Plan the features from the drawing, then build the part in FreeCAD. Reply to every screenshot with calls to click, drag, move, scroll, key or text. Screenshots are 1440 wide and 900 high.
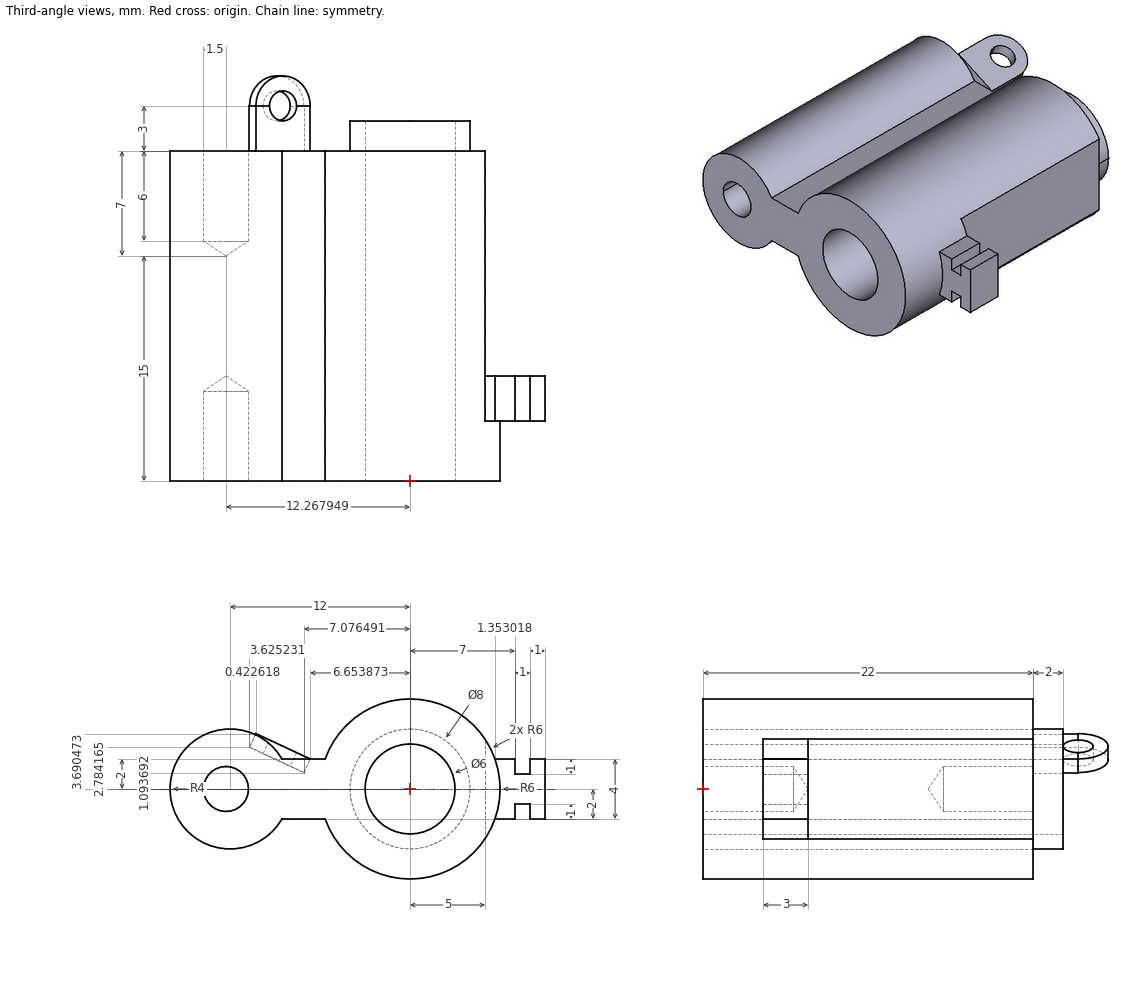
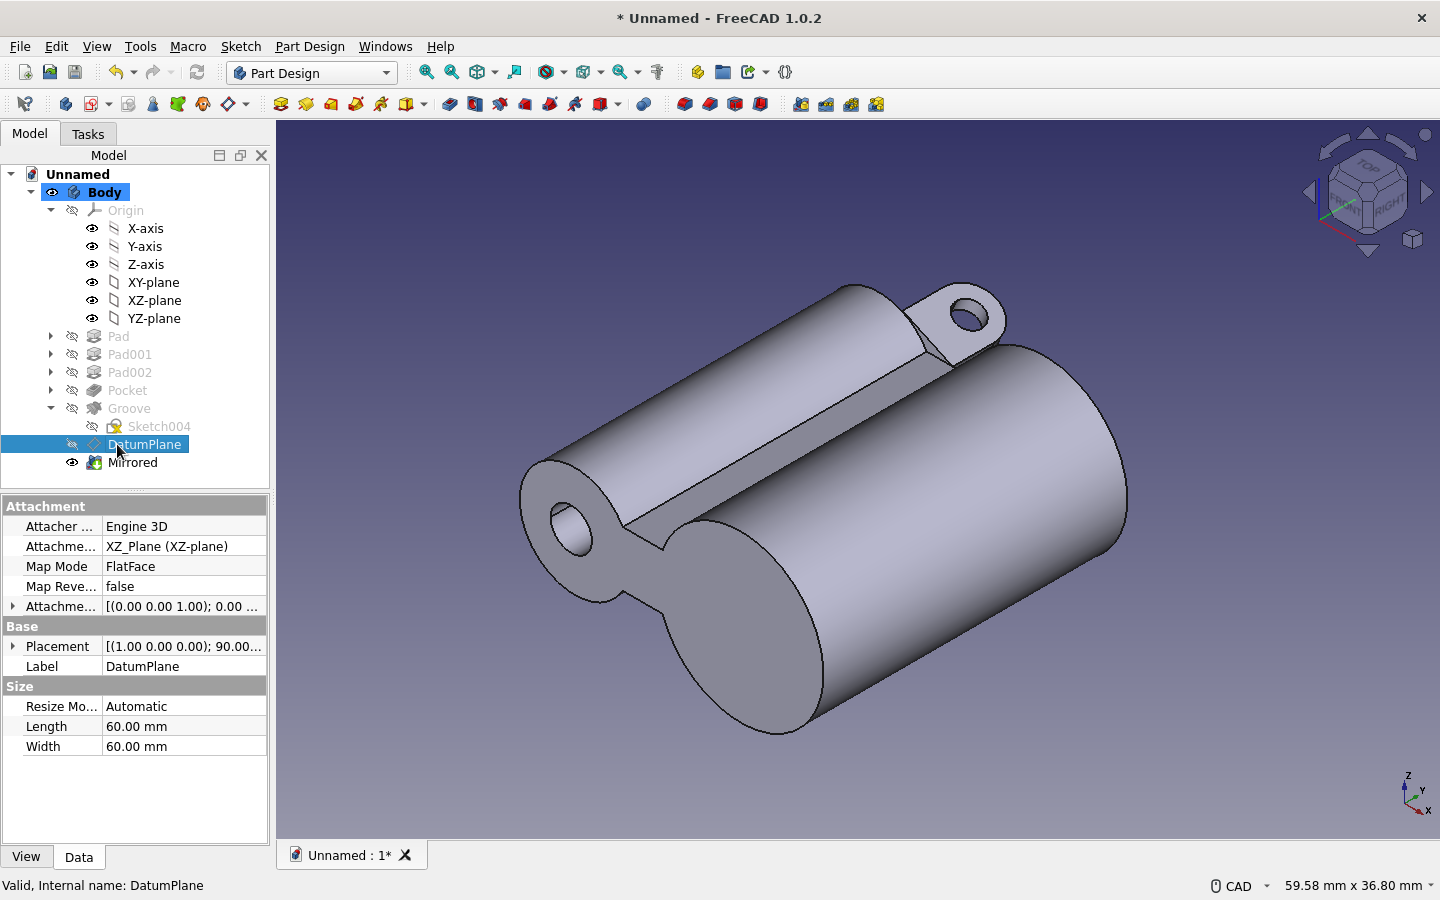
key(4)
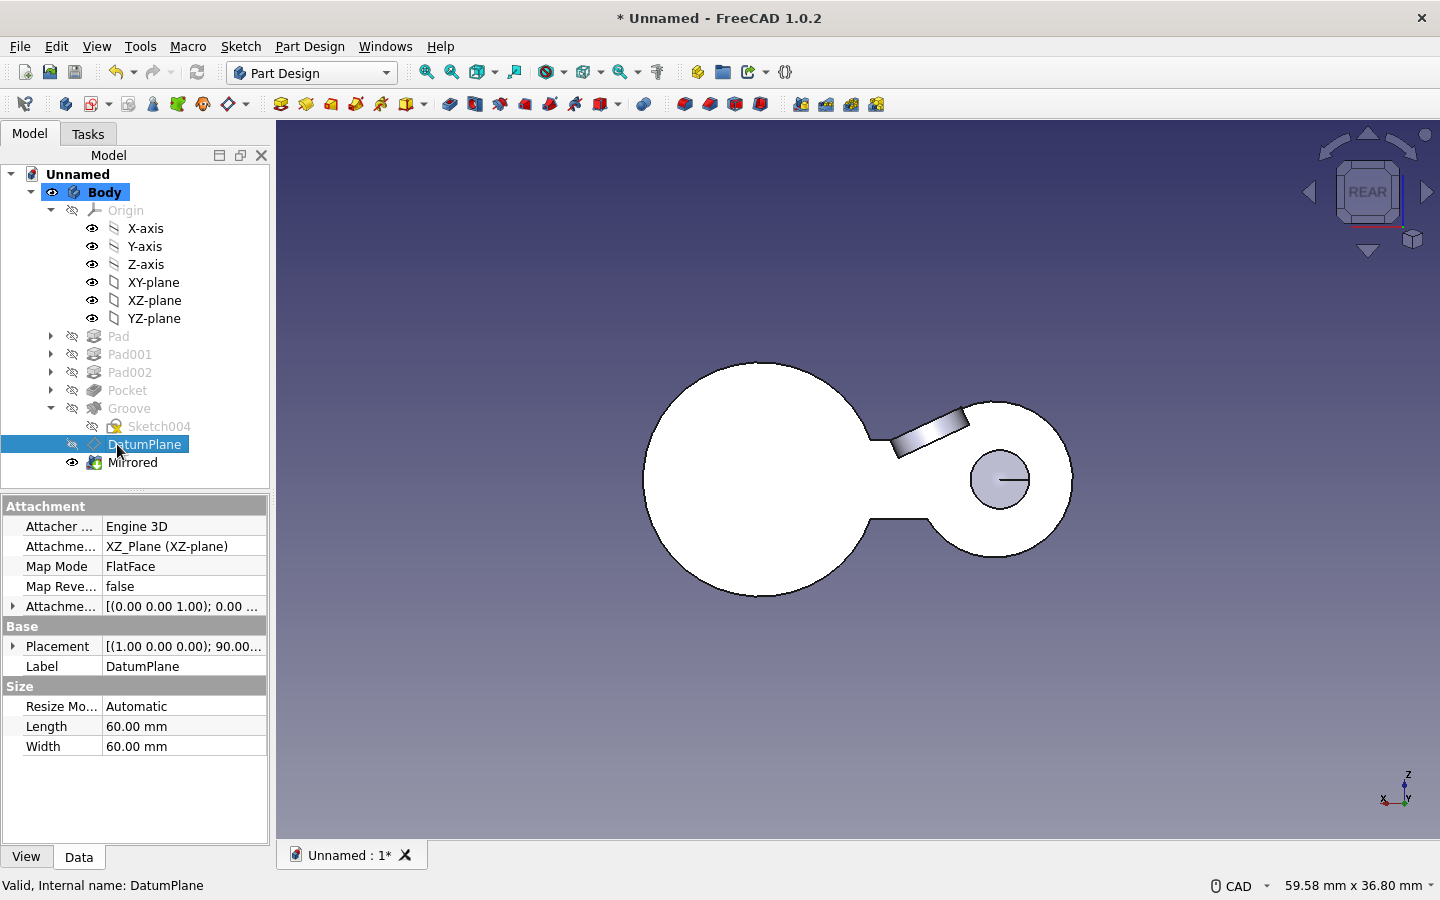
click(427, 72)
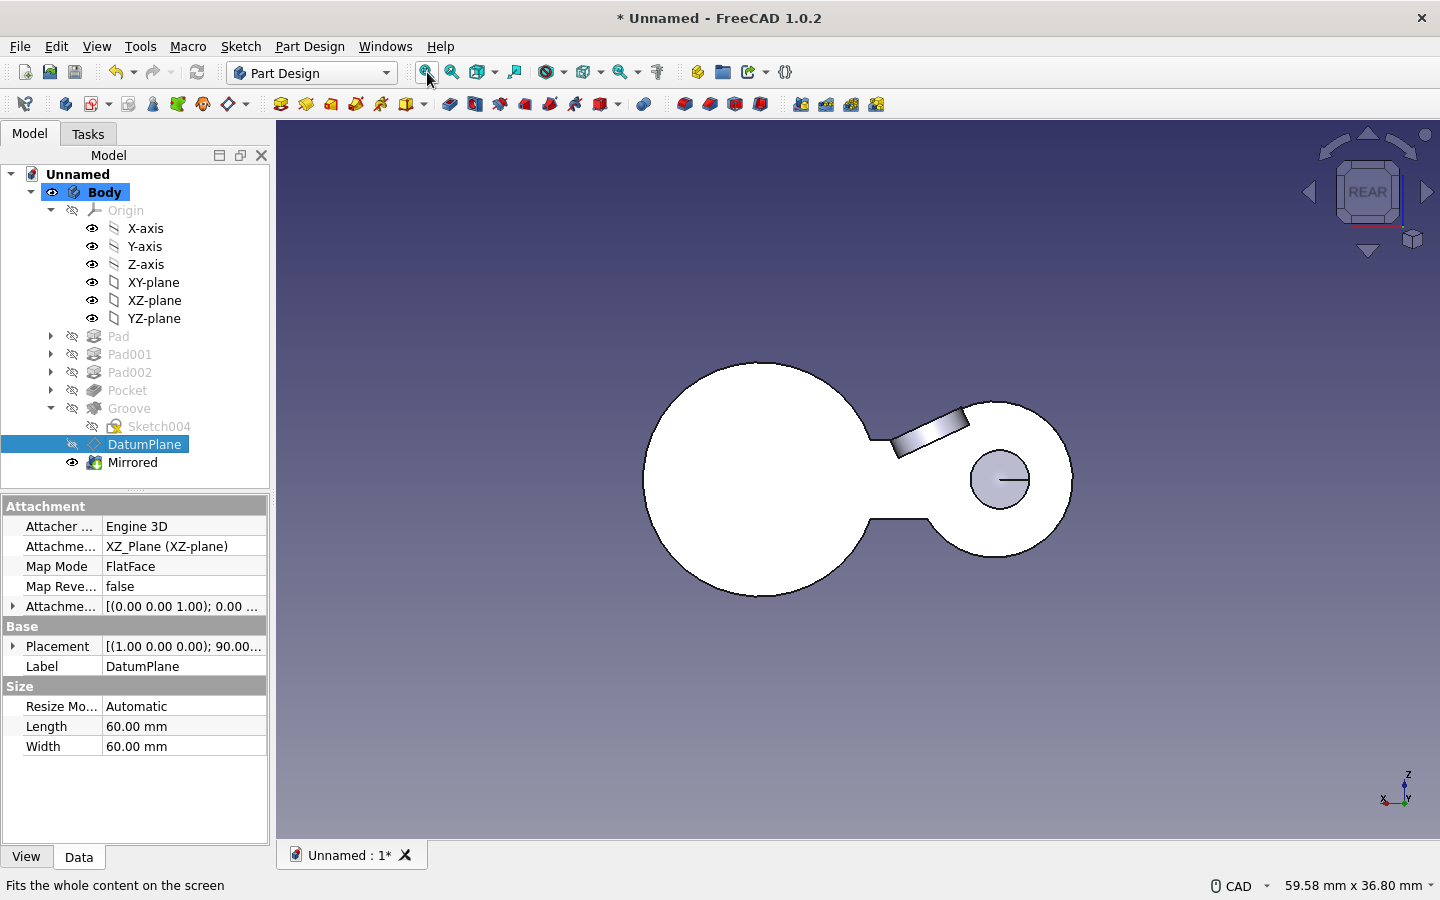
click(735, 479)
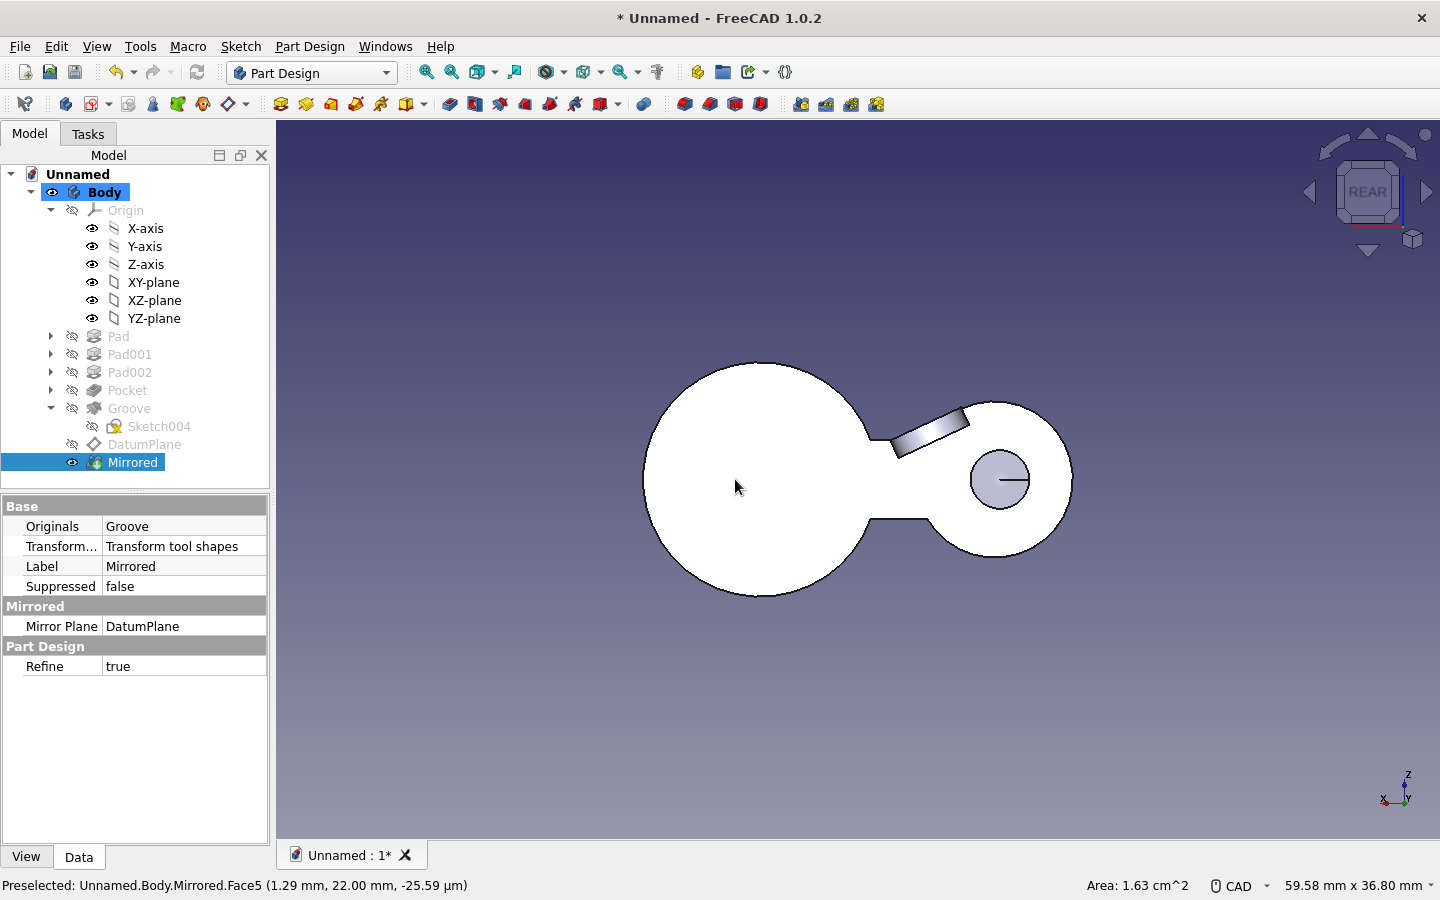
click(90, 104)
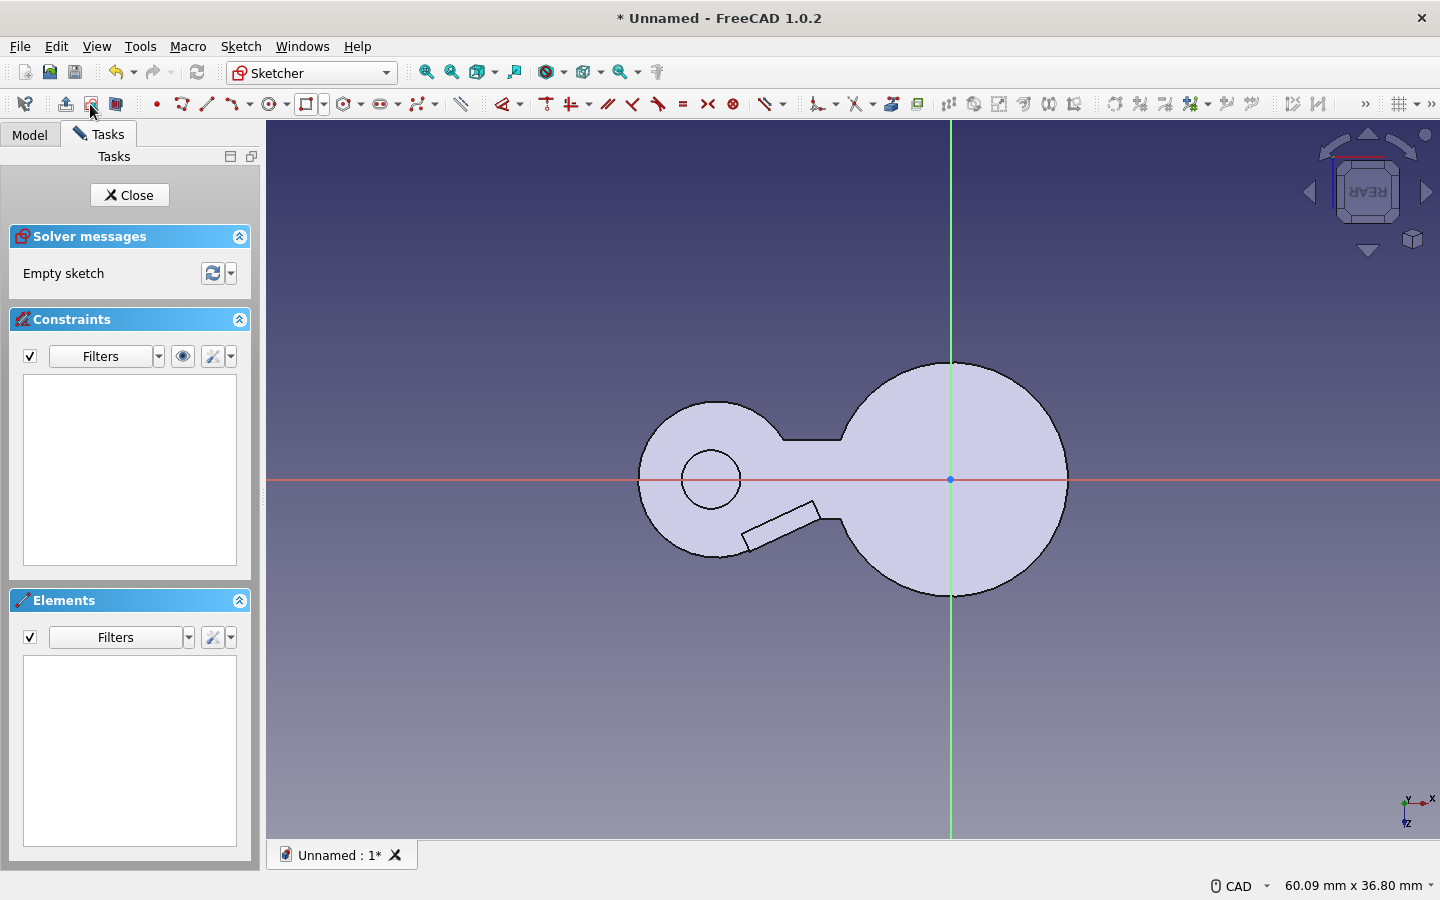
click(116, 104)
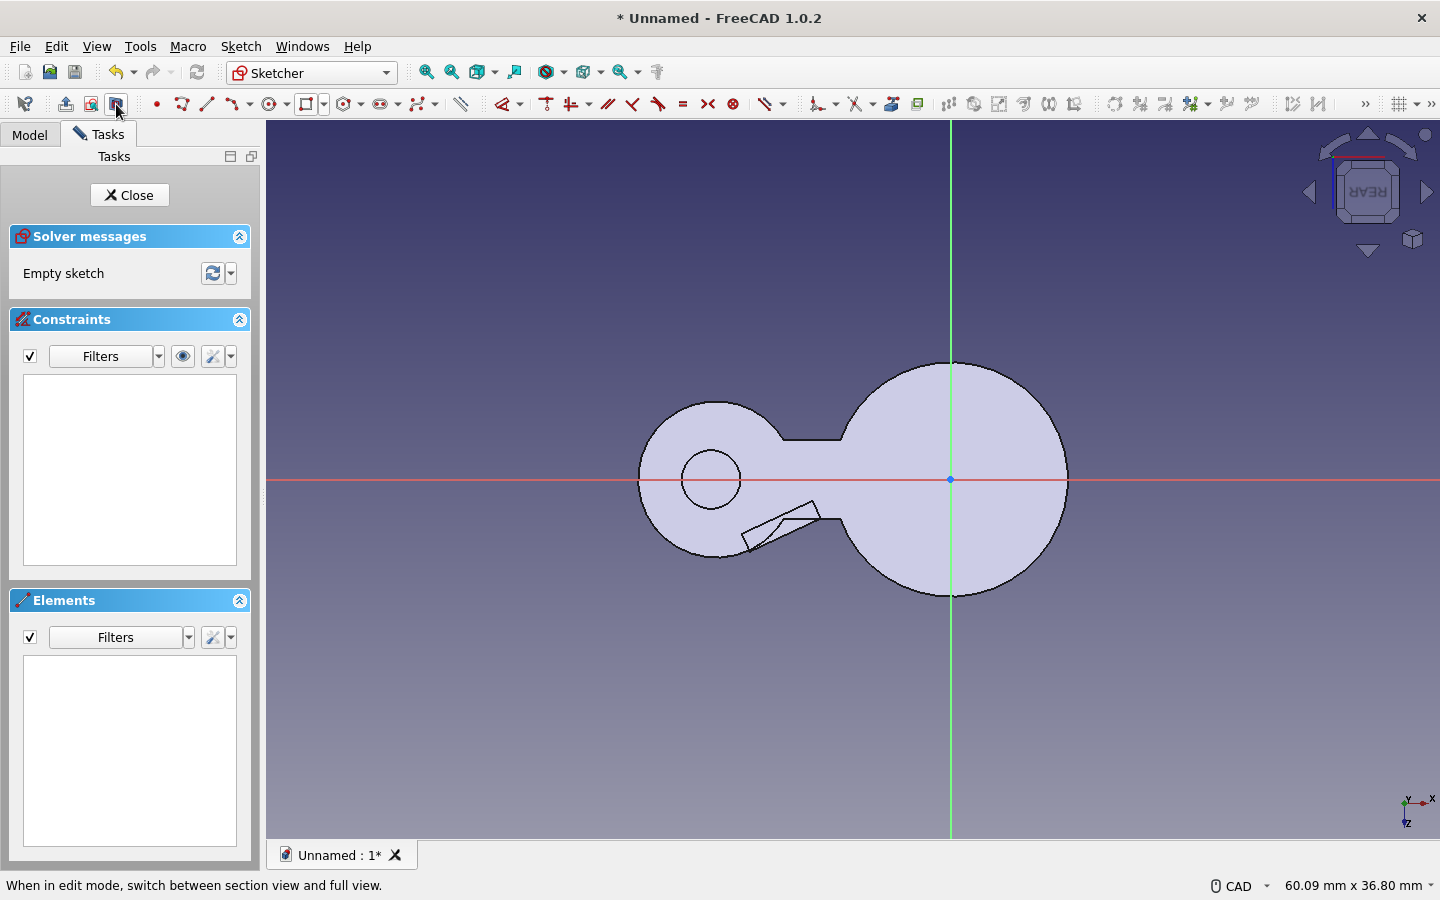
scroll(1047, 479, up, 5)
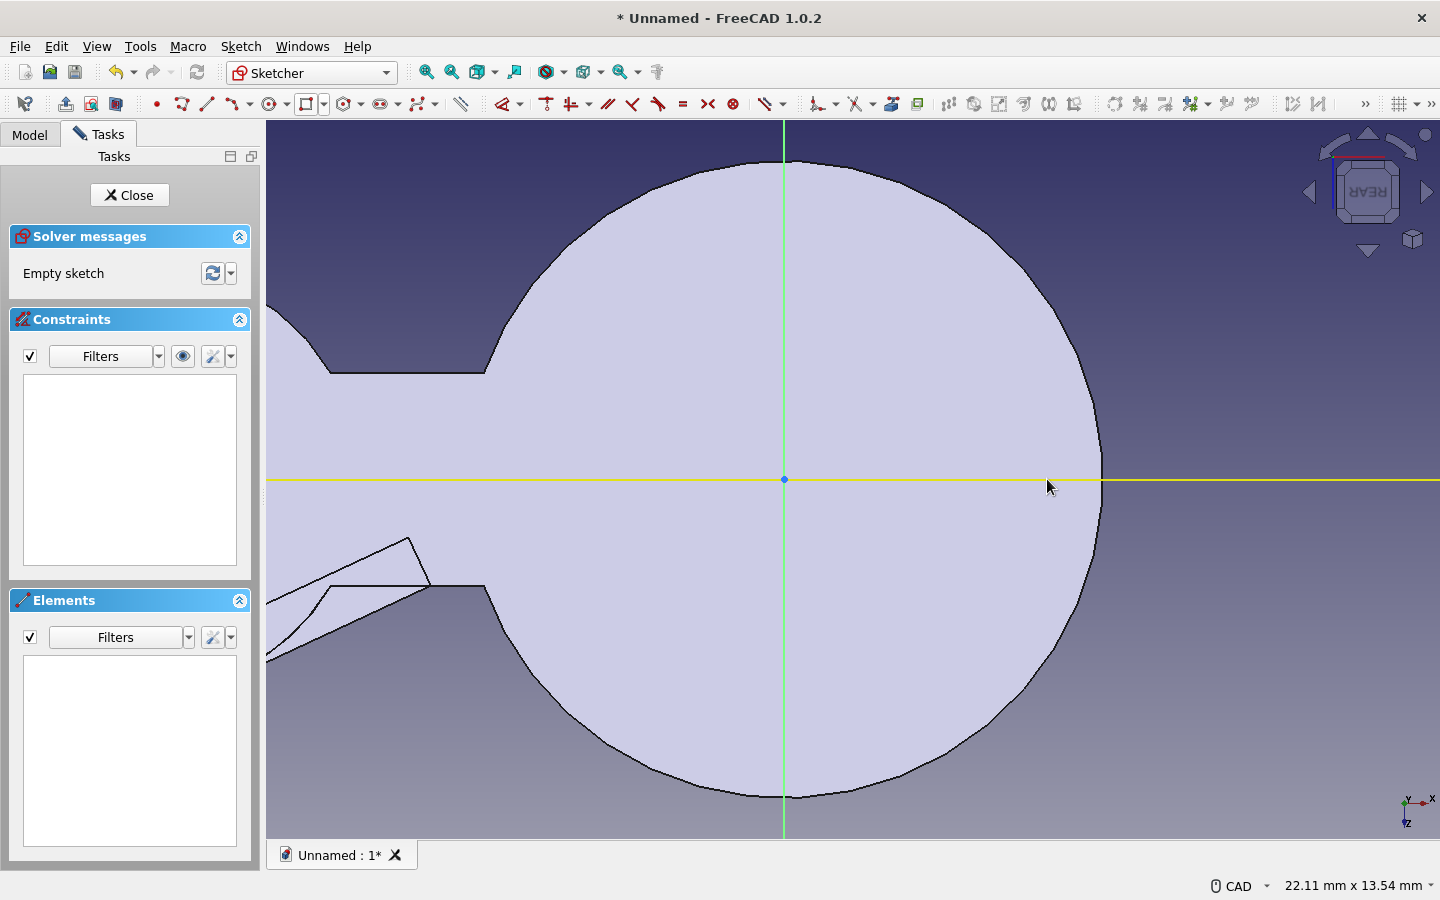
click(268, 104)